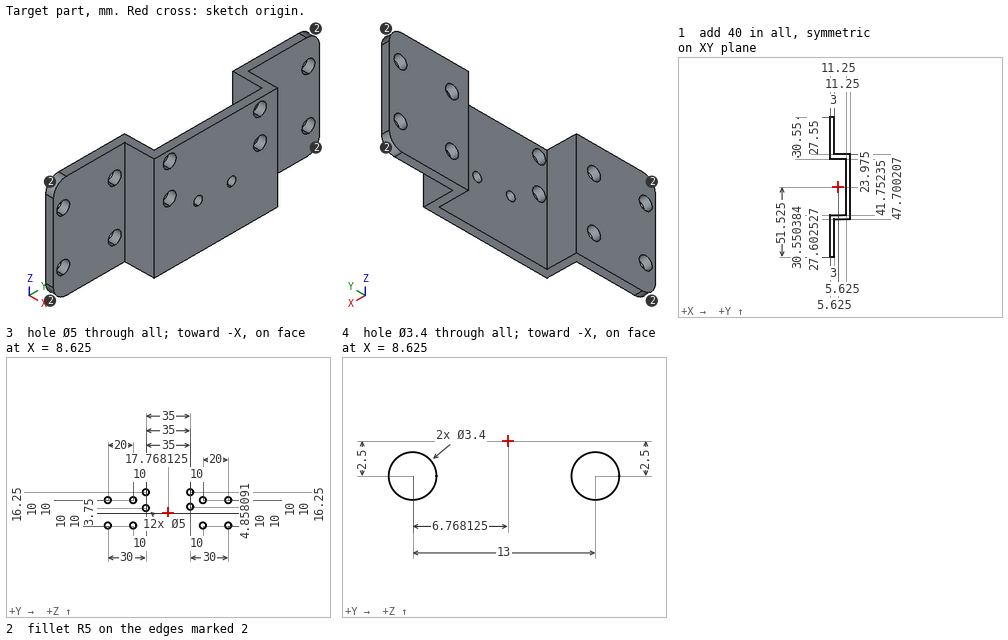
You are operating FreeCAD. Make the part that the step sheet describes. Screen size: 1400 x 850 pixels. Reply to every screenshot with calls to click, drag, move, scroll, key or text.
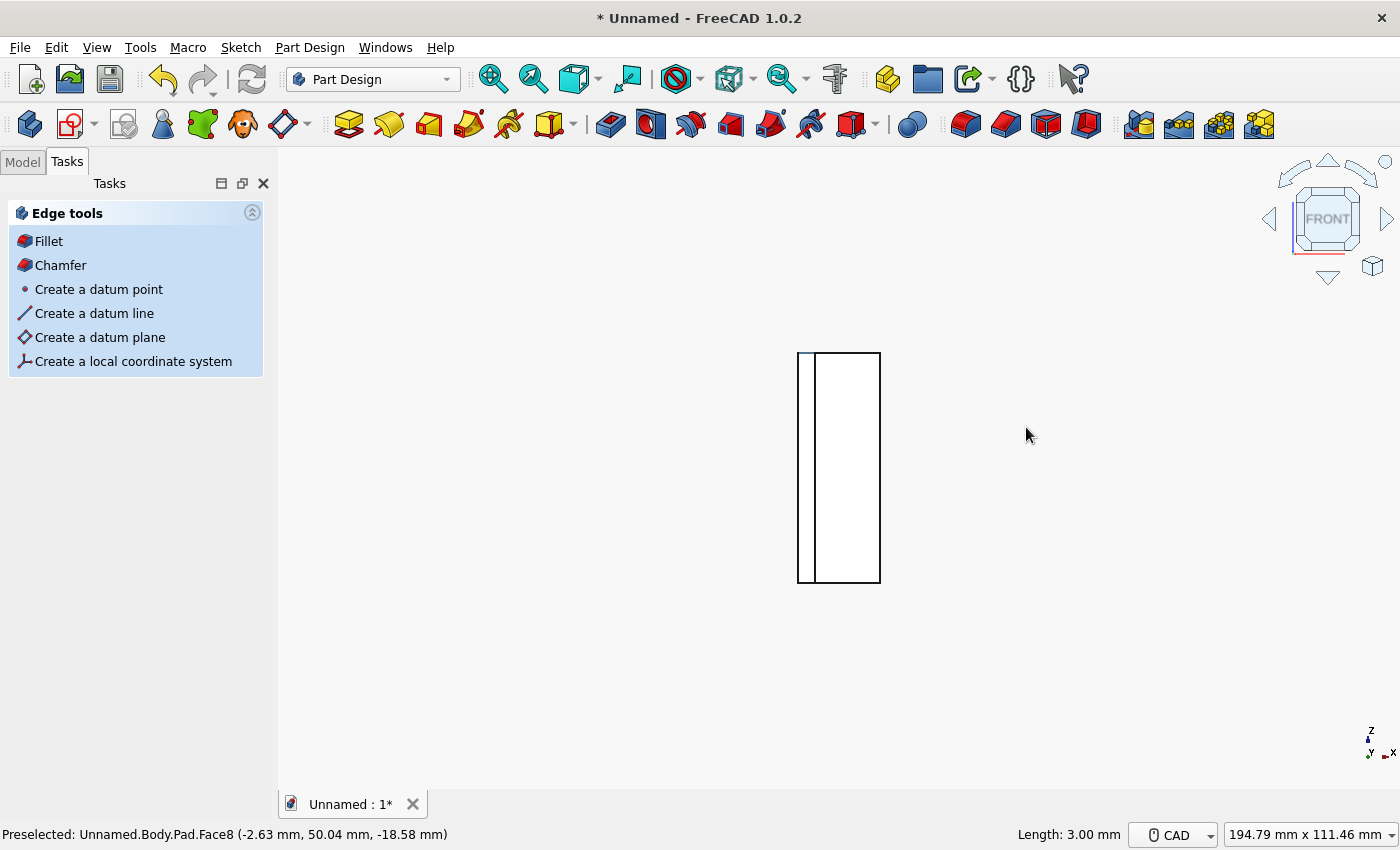
click(494, 80)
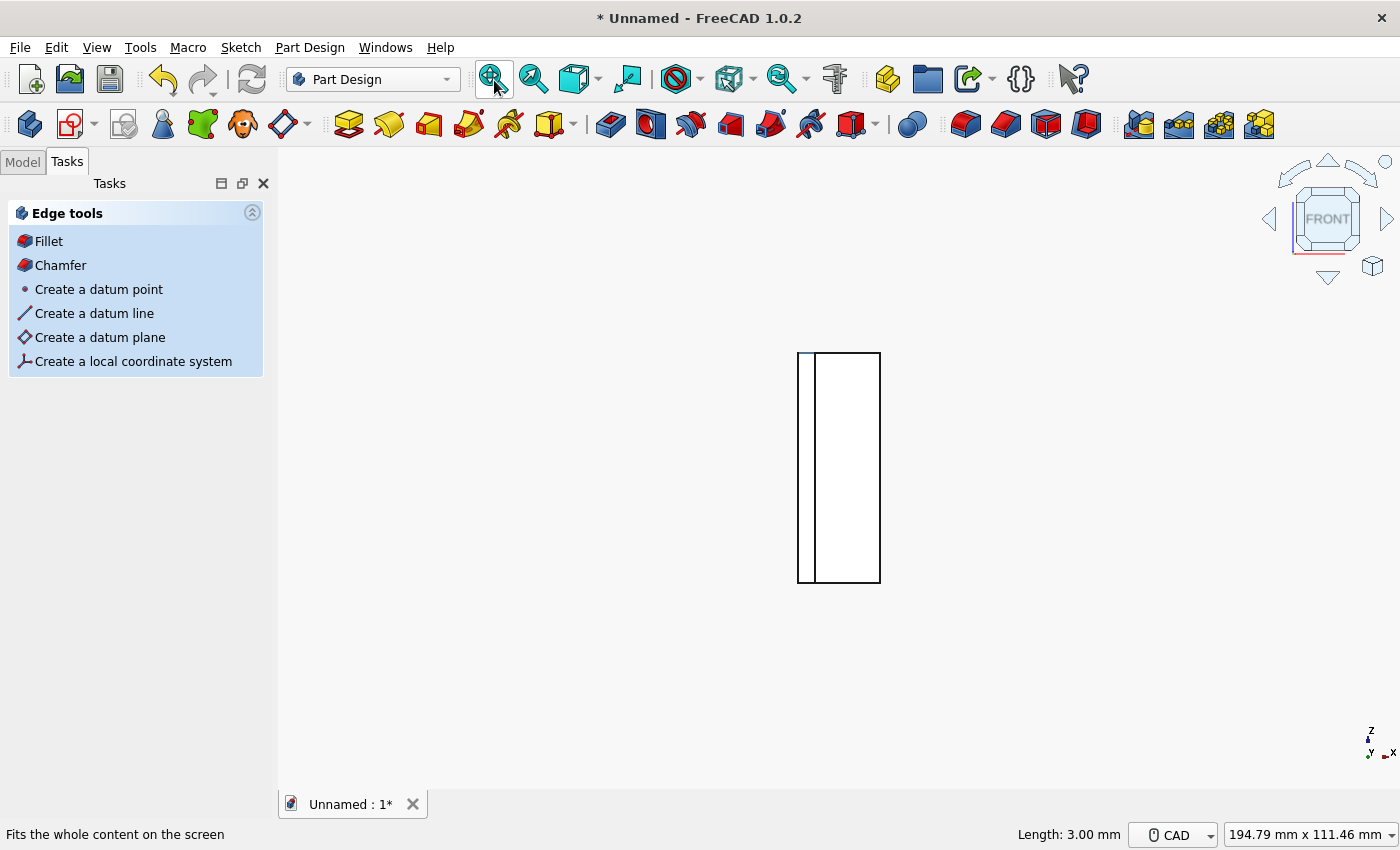
click(807, 582, ctrl)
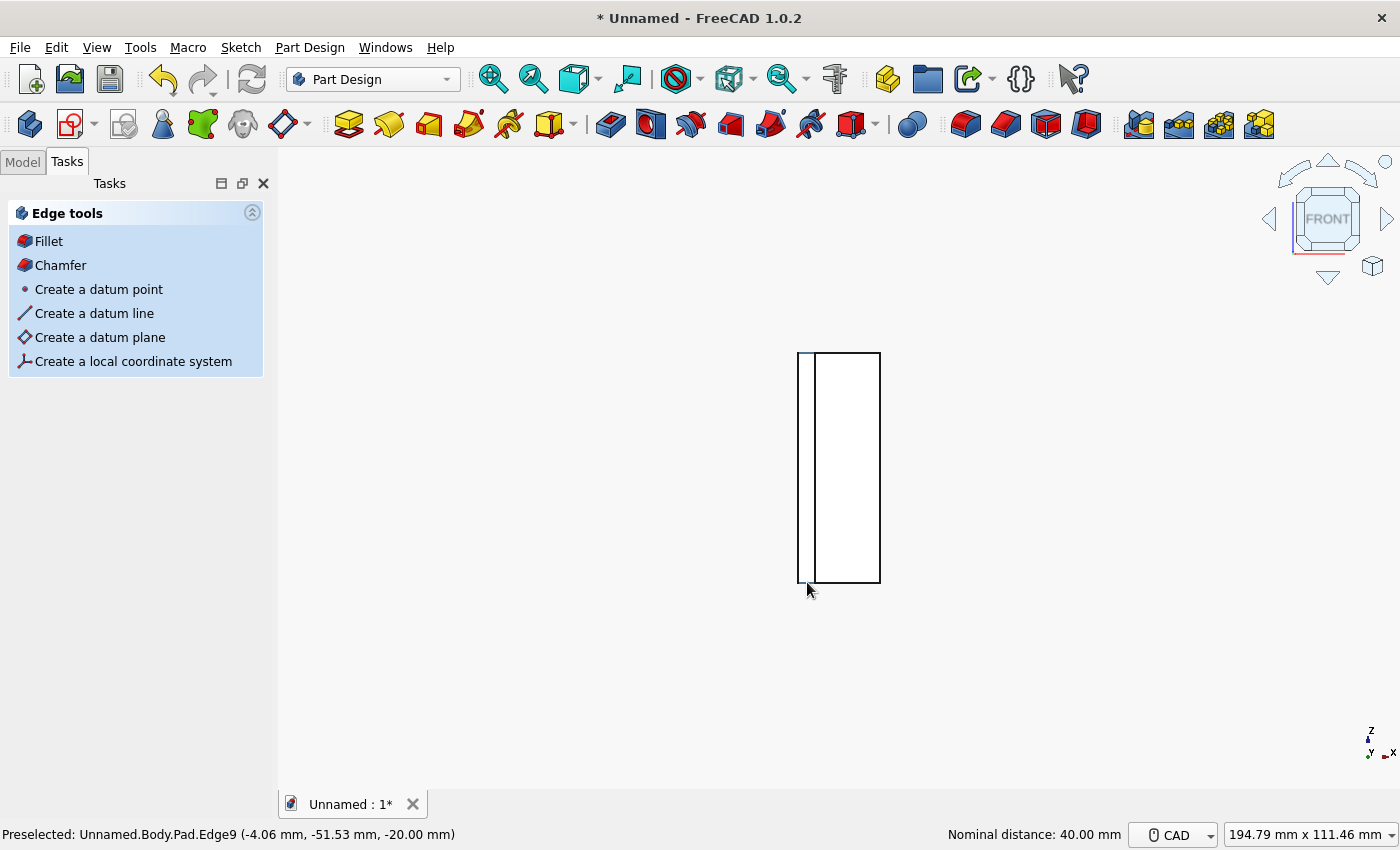
scroll(807, 582, up, 5)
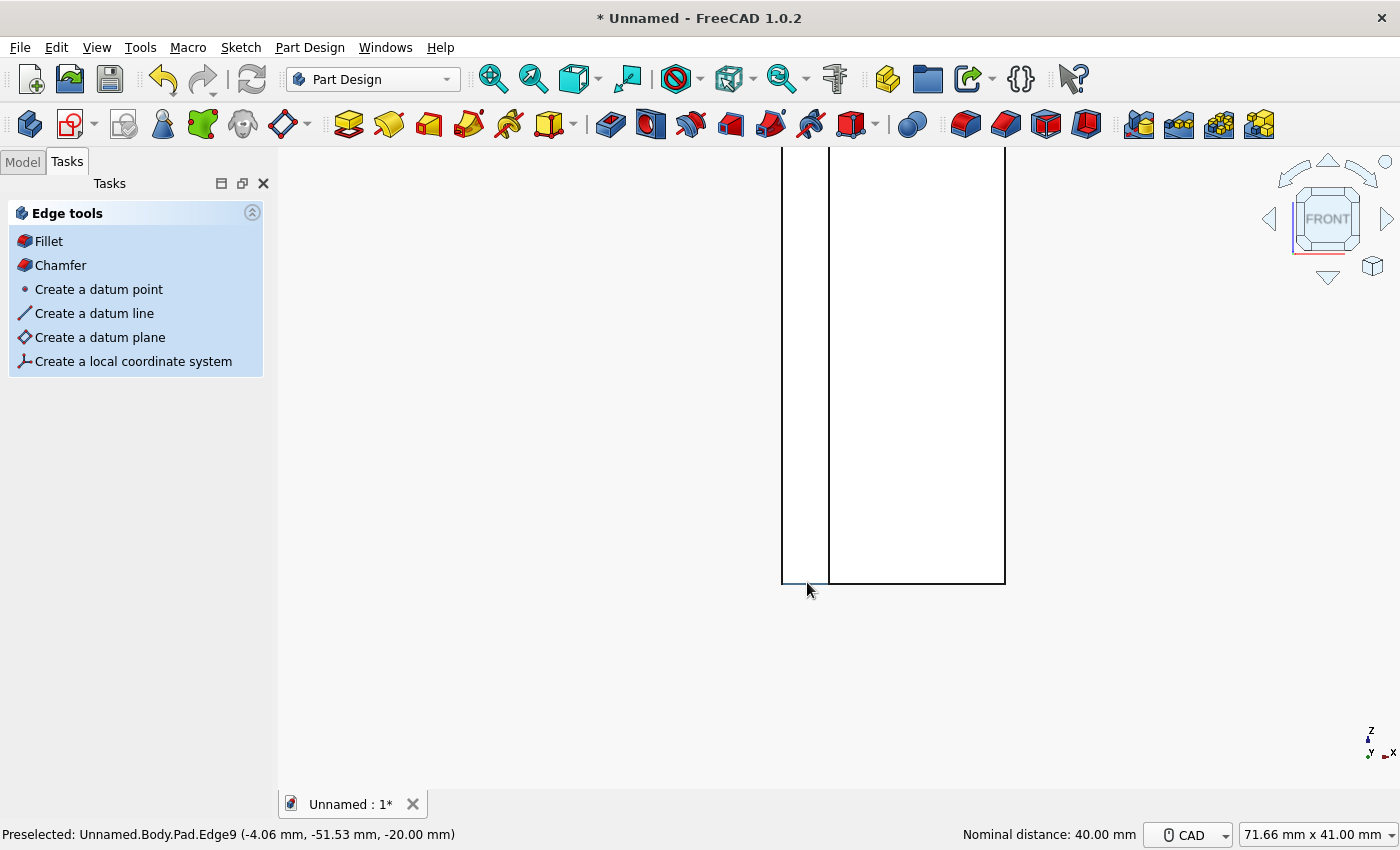
click(494, 80)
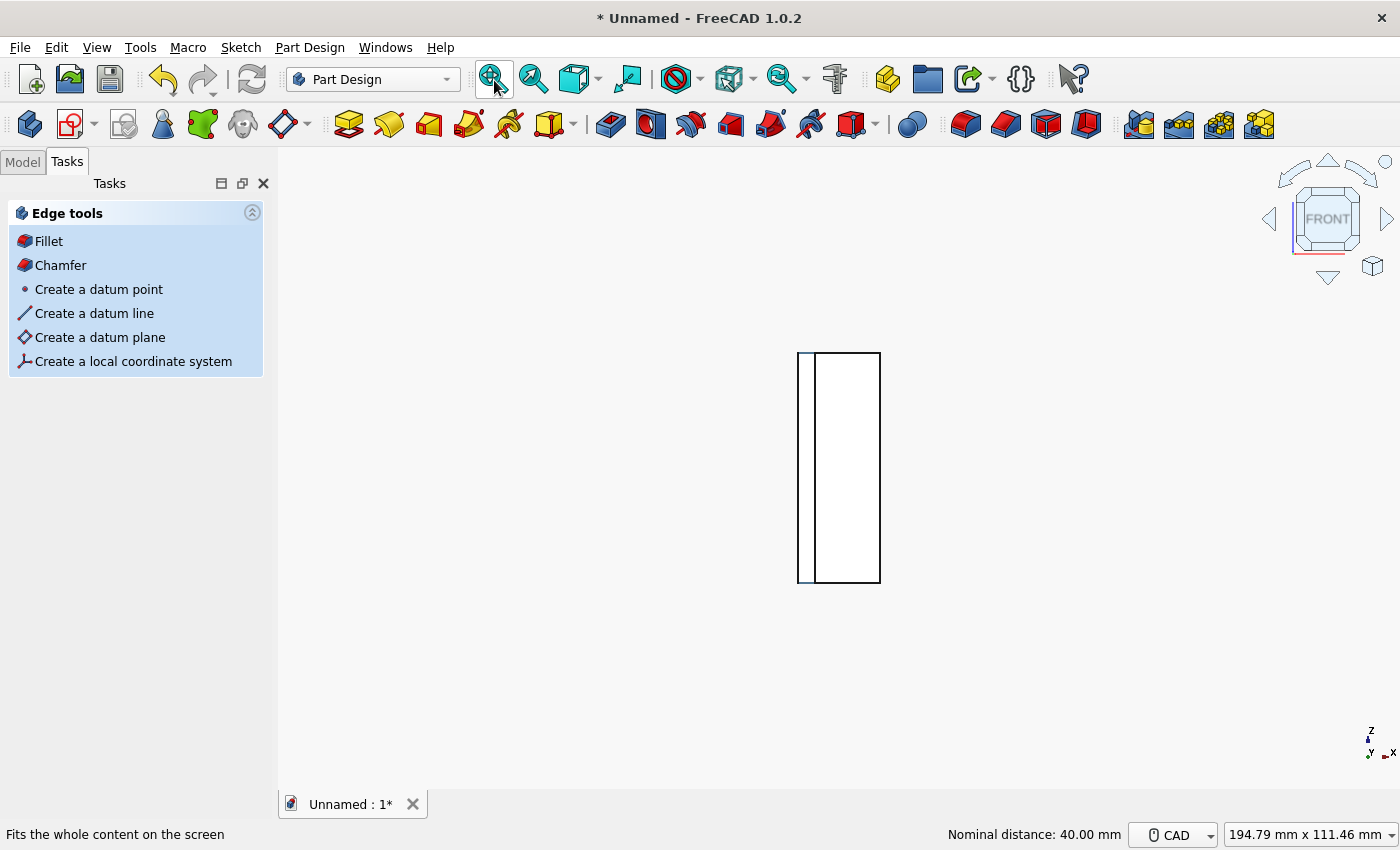
key(3)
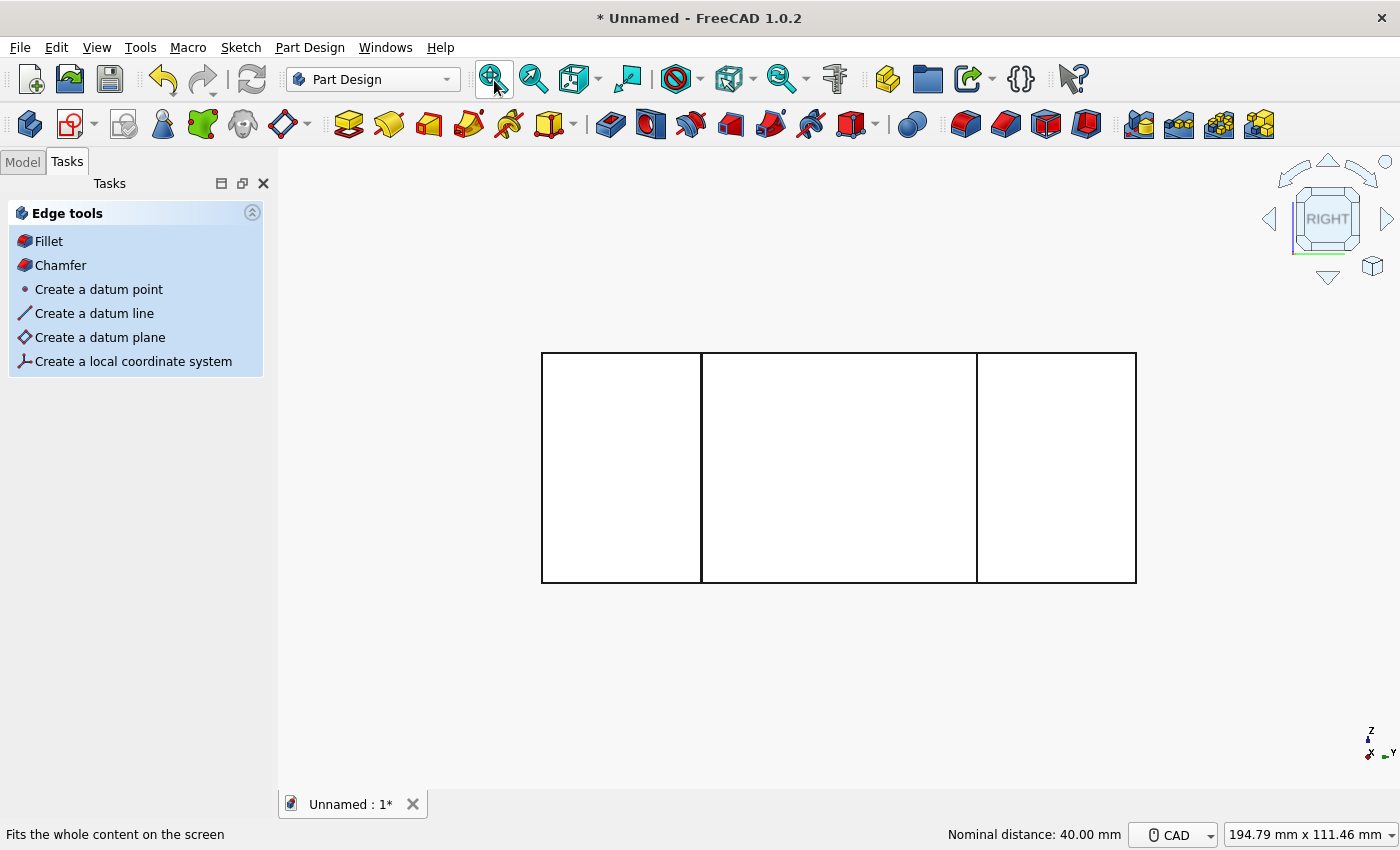
scroll(1136, 582, up, 5)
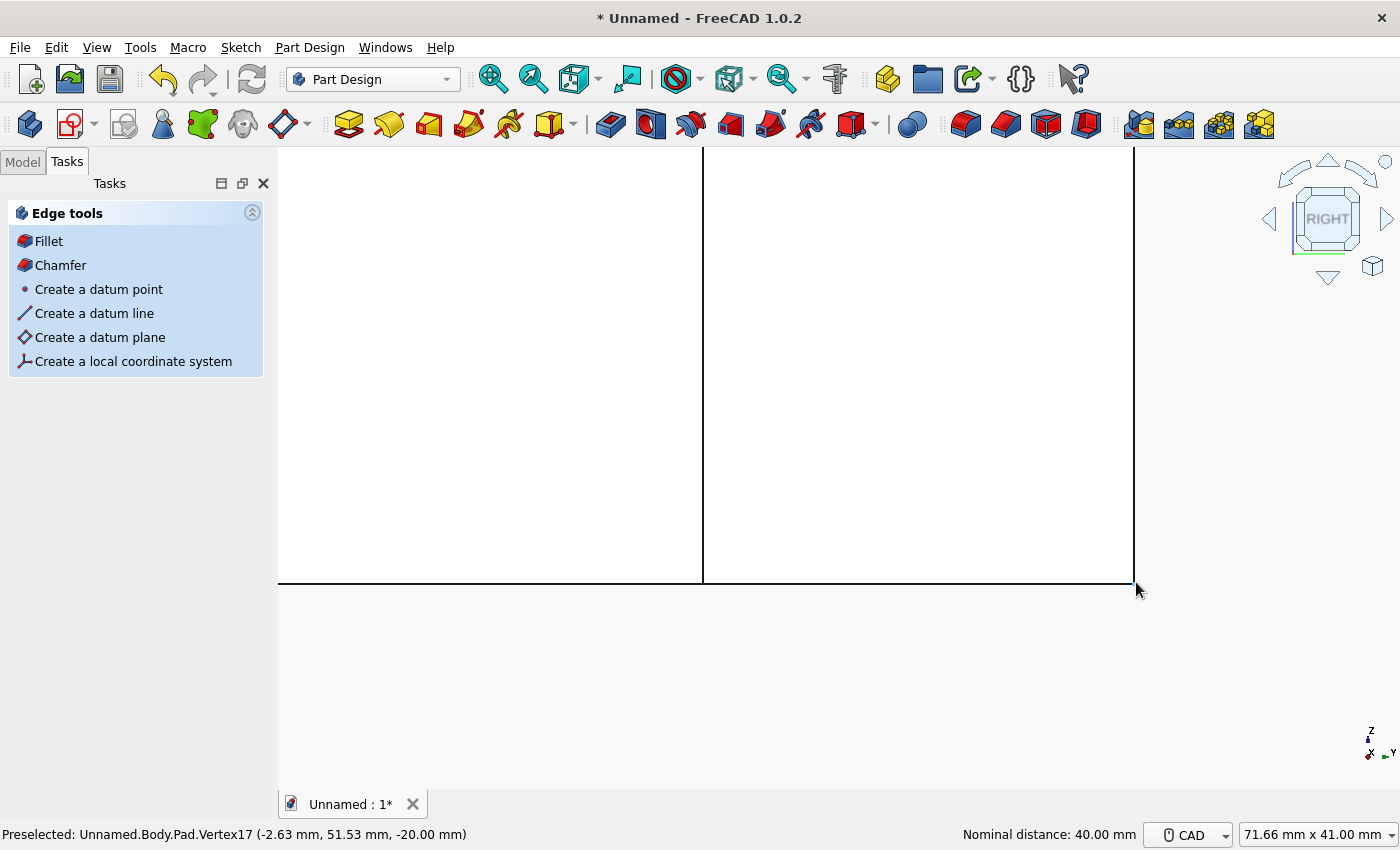
click(494, 80)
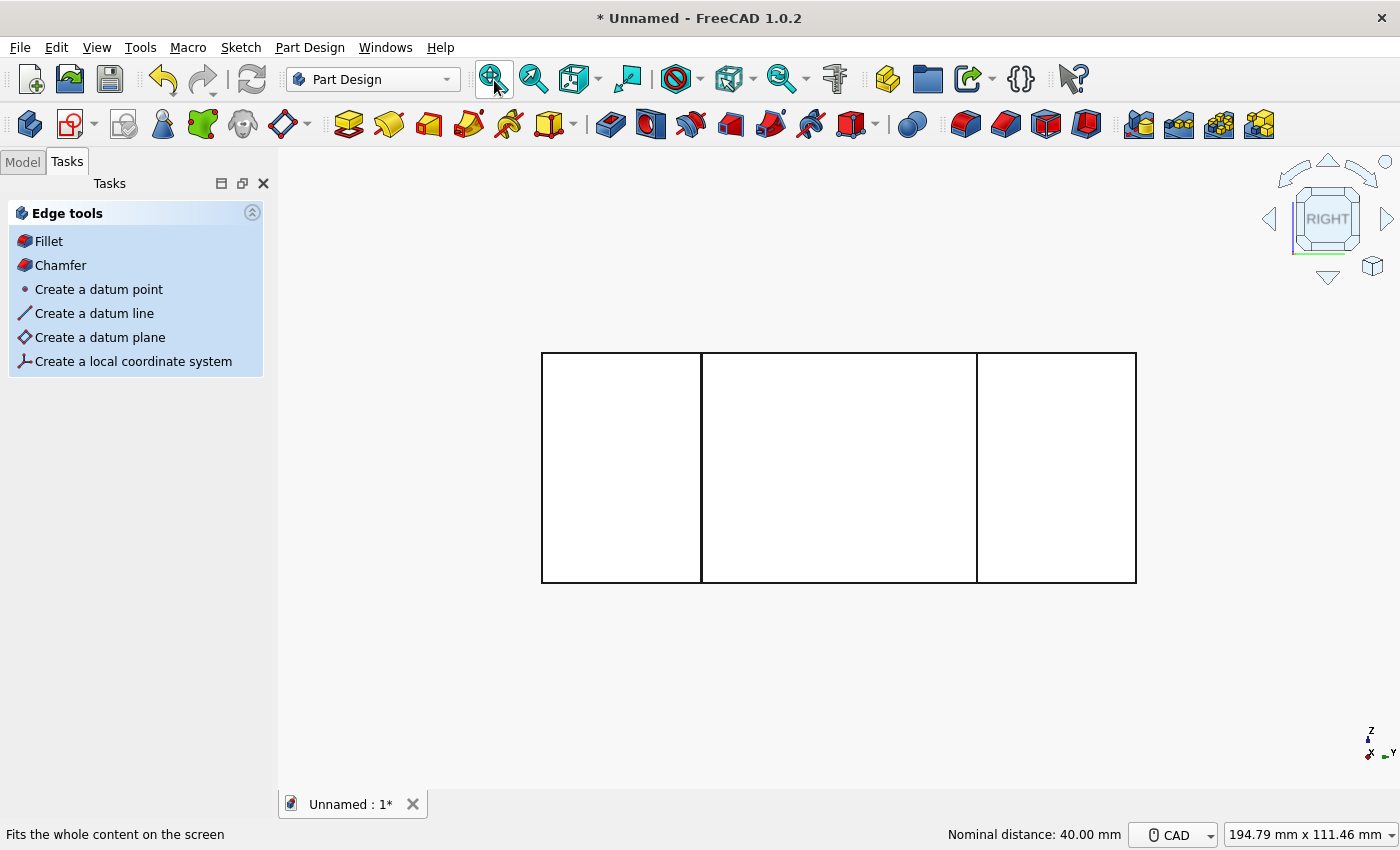
key(5)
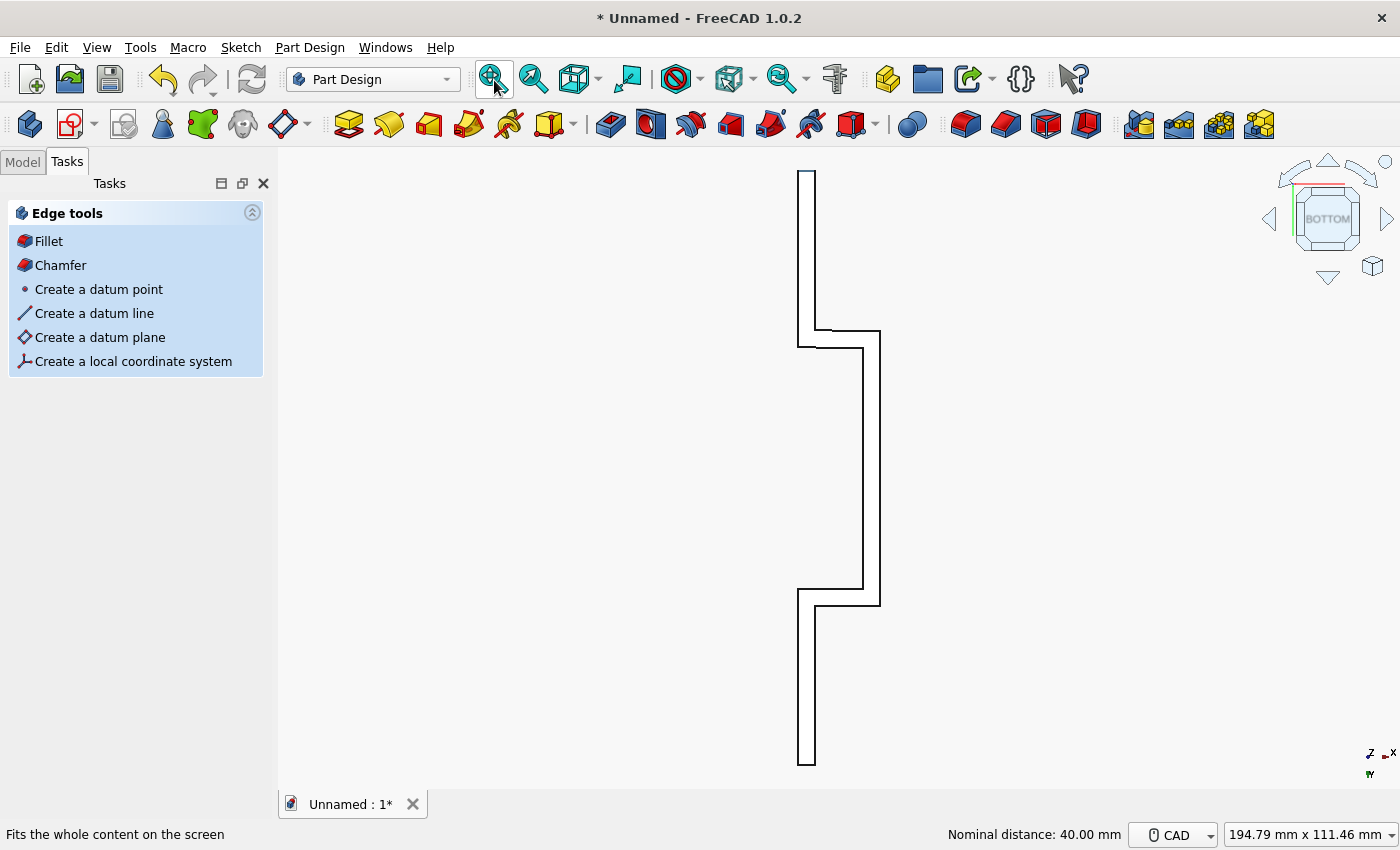
key(4)